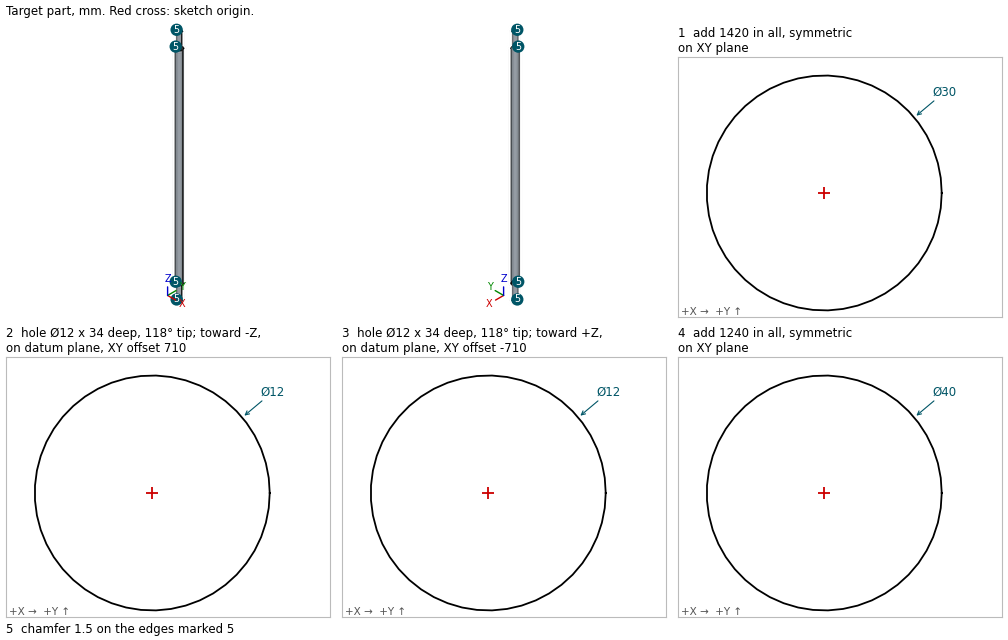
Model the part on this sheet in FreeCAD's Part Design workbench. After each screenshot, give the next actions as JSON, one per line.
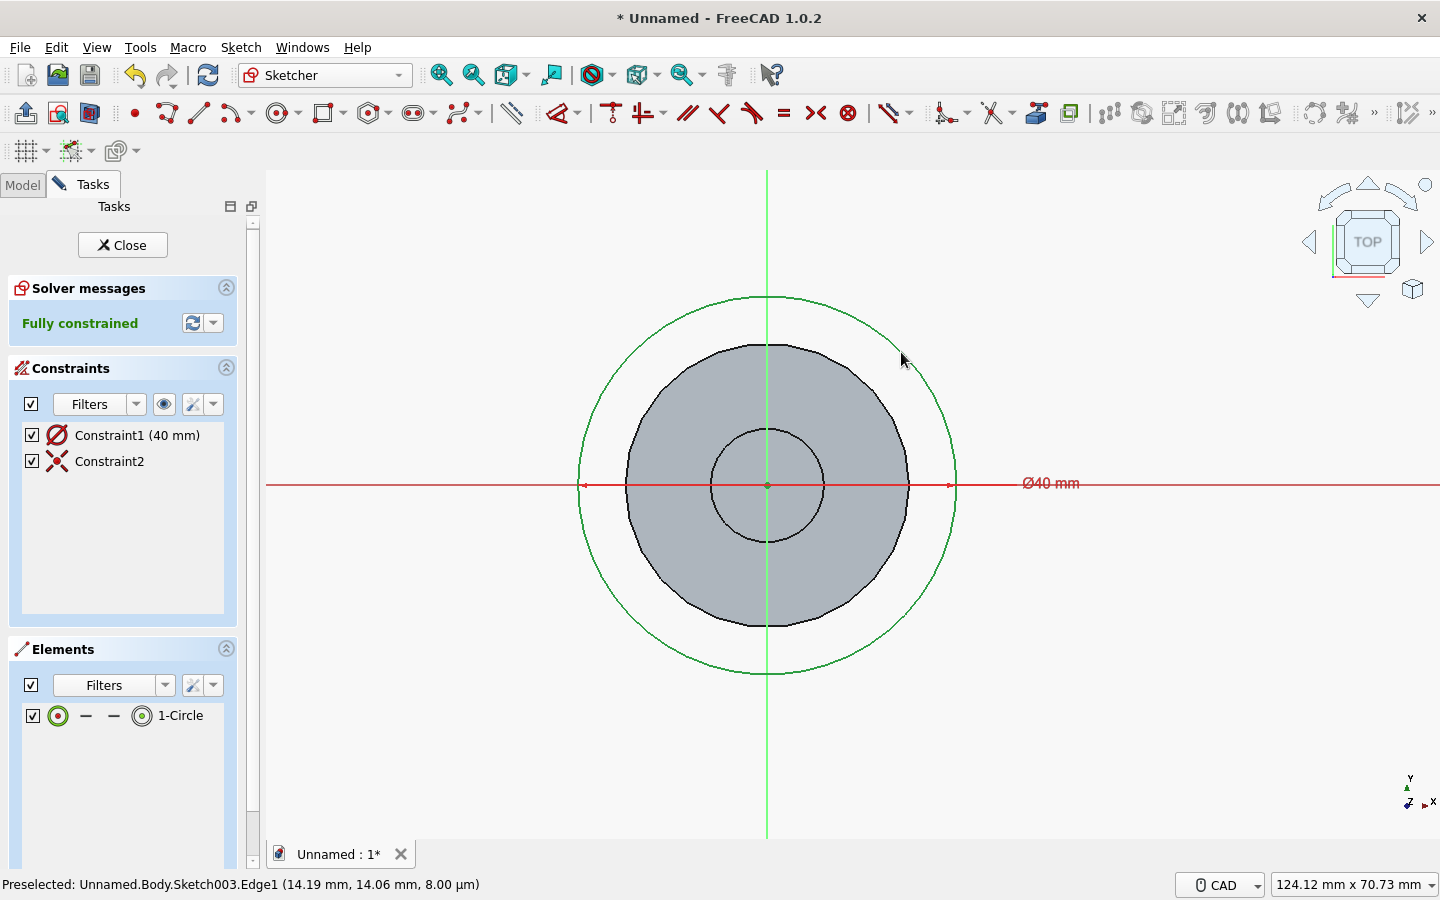
{"action": "left_click", "coordinate": [123, 245]}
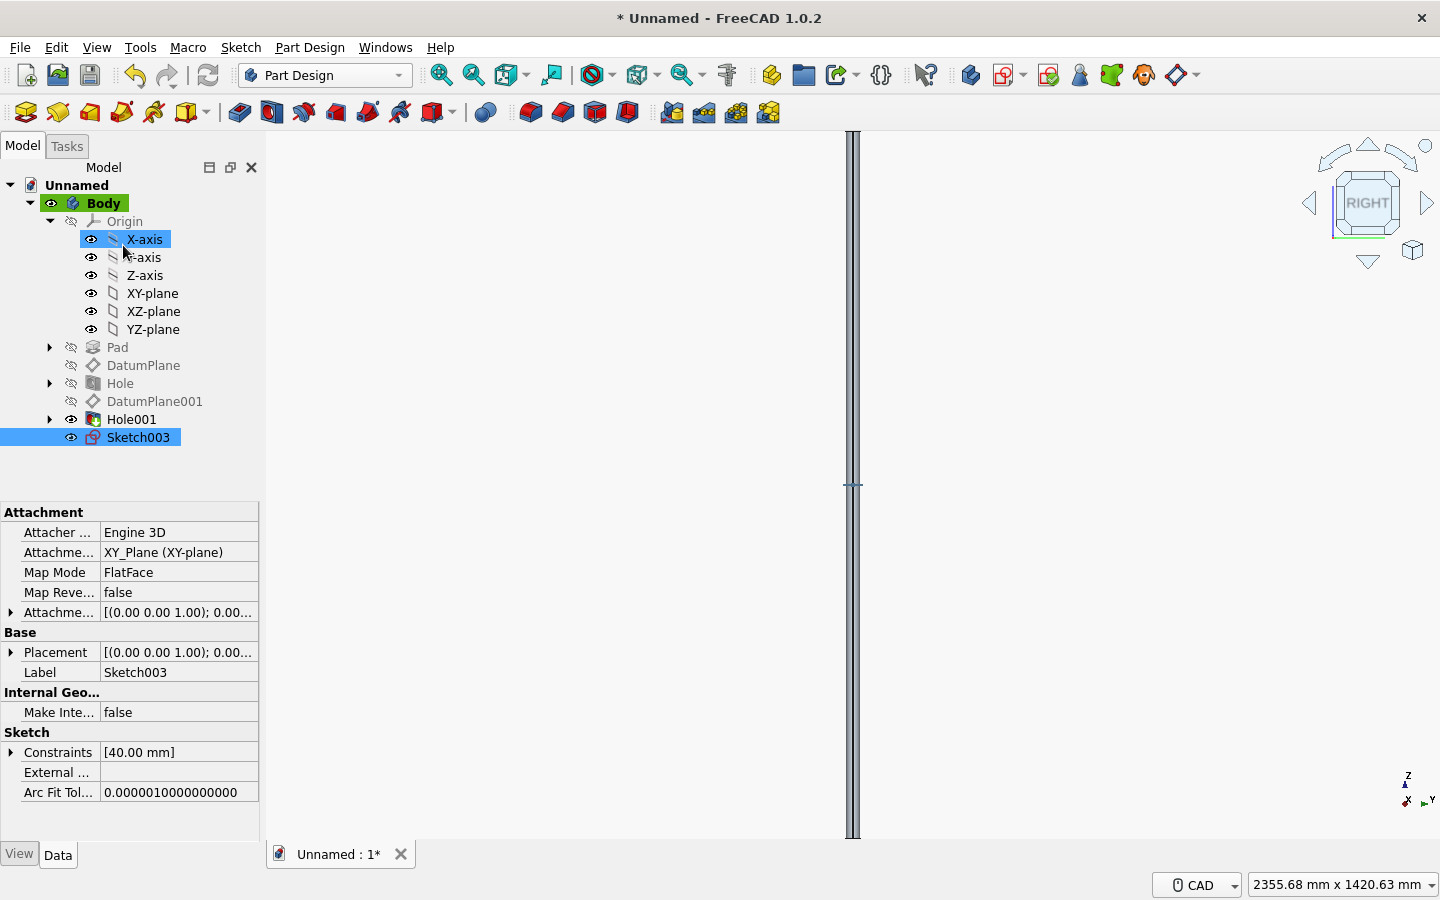
{"action": "left_click", "coordinate": [26, 112]}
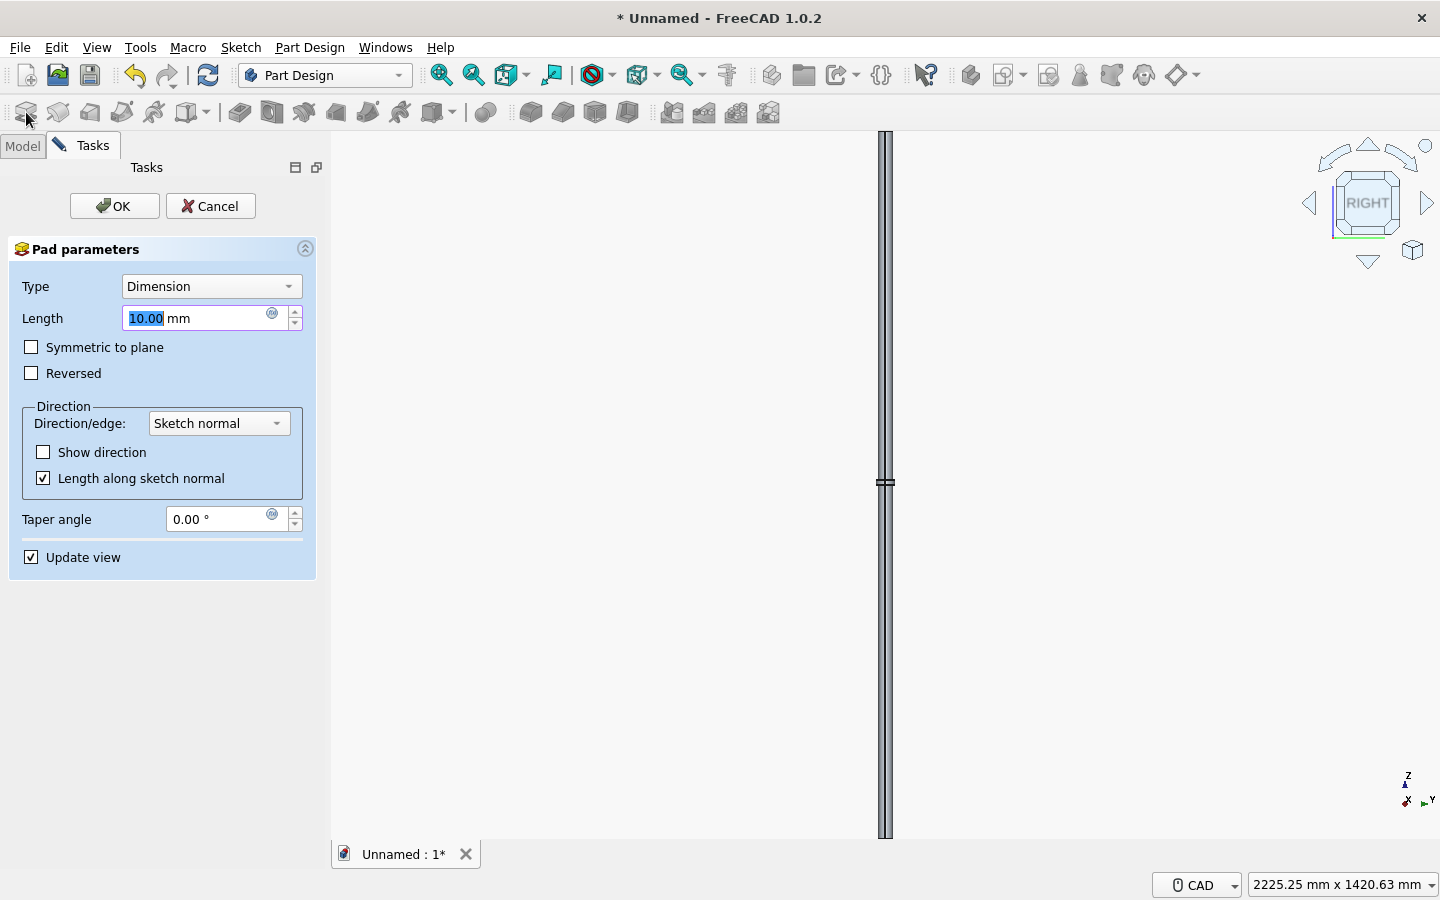
{"action": "type", "text": "1240"}
{"action": "key", "text": "Tab"}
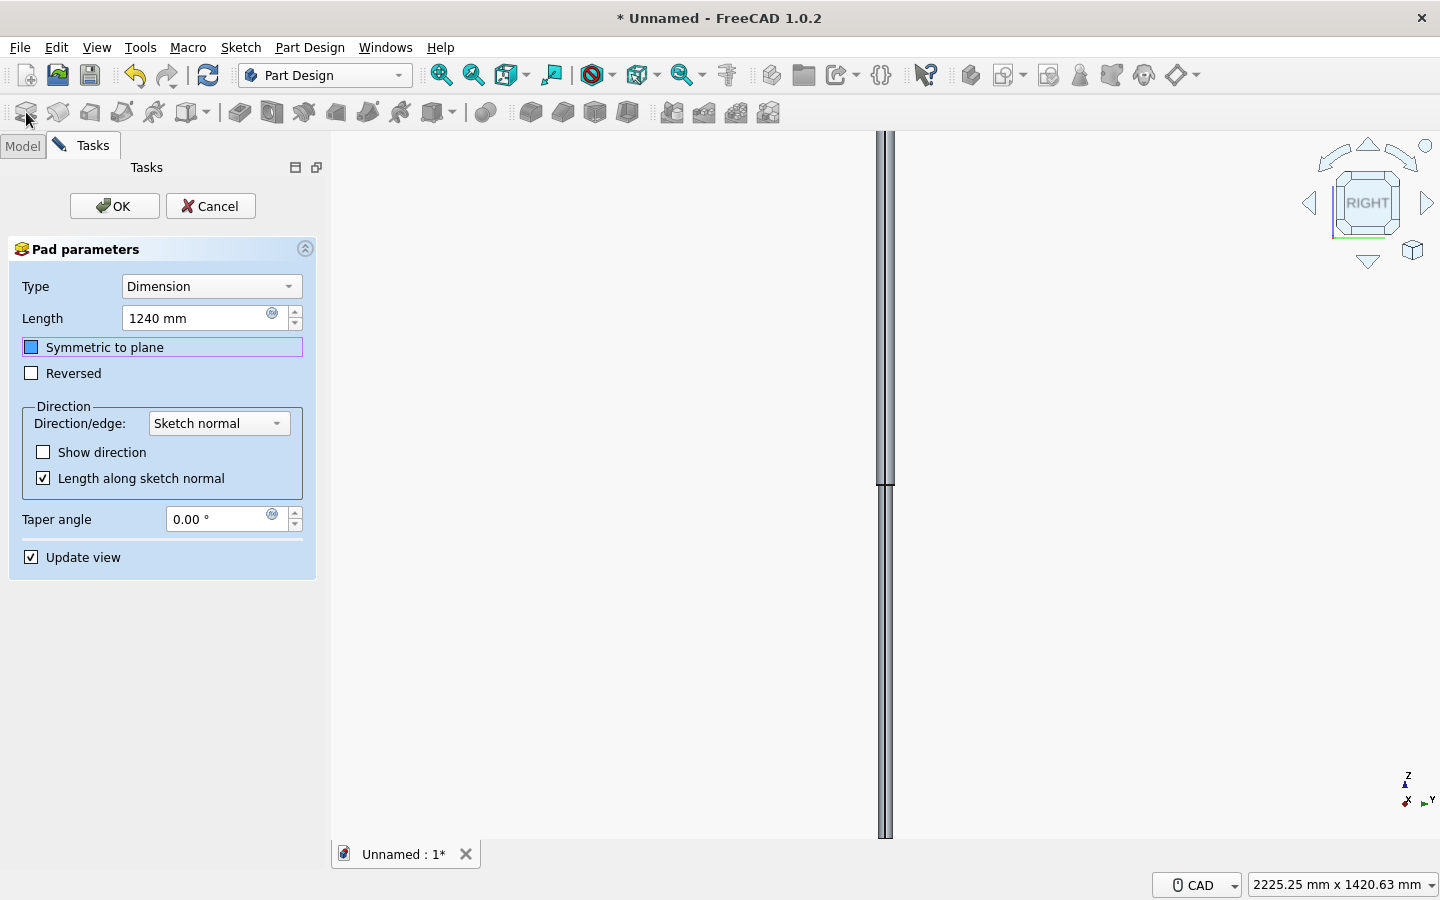
{"action": "left_click", "coordinate": [30, 347]}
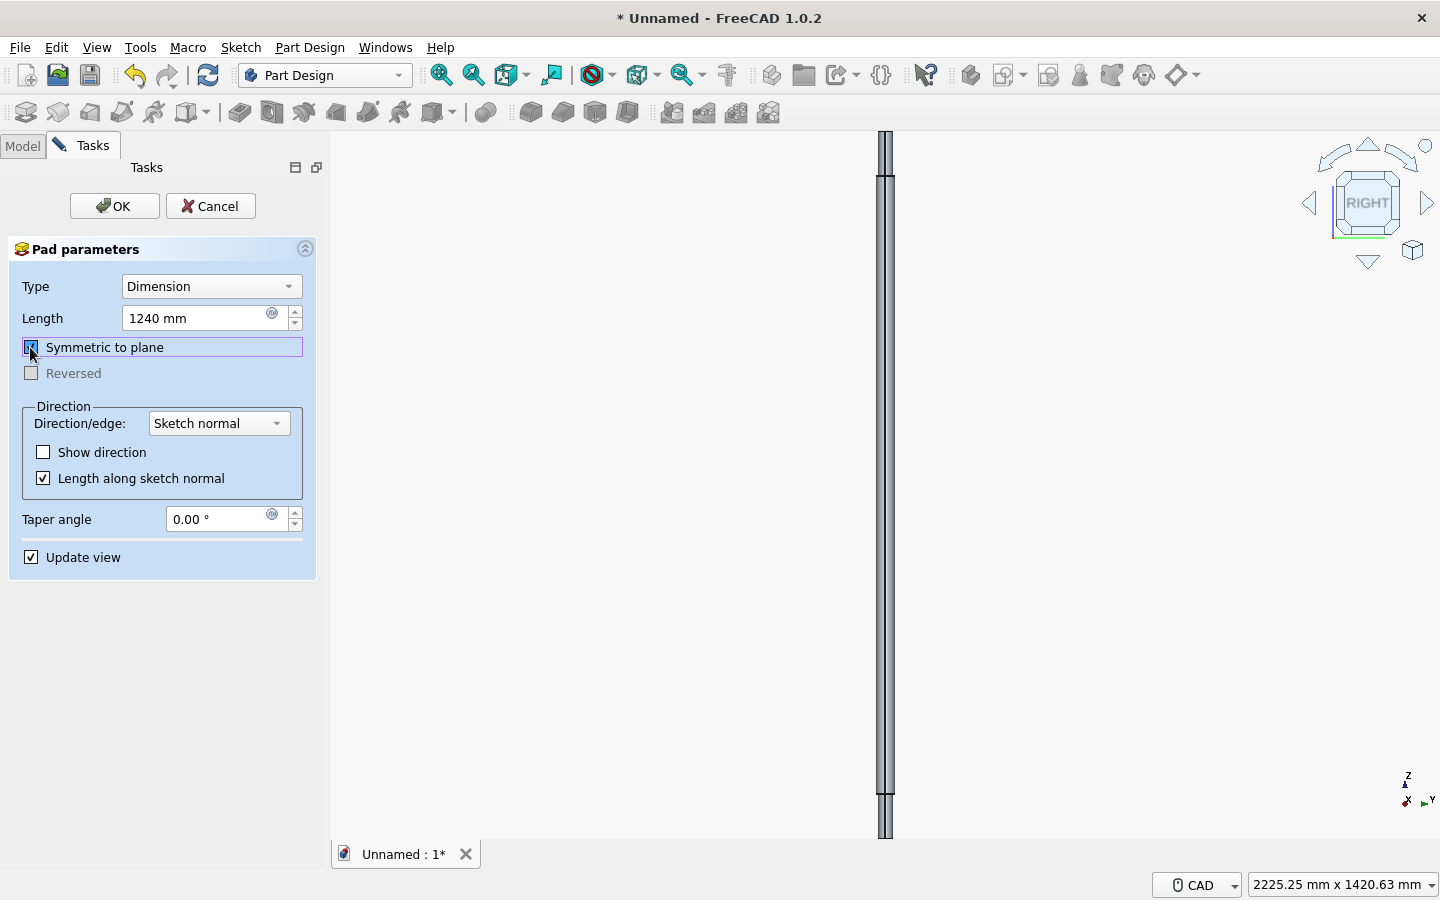
{"action": "left_click", "coordinate": [115, 206]}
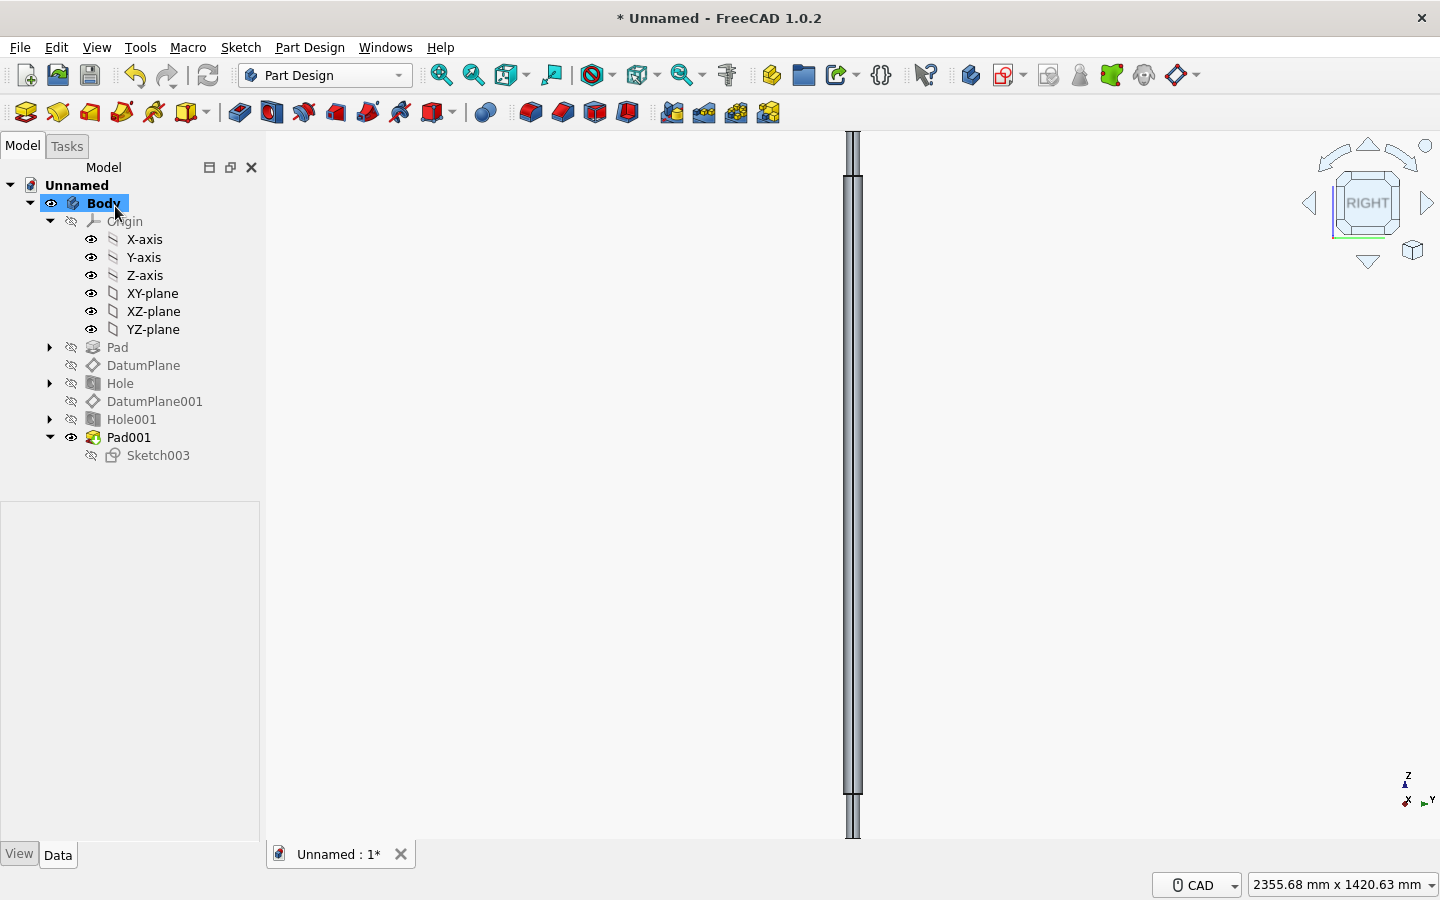
{"action": "left_click", "coordinate": [442, 76]}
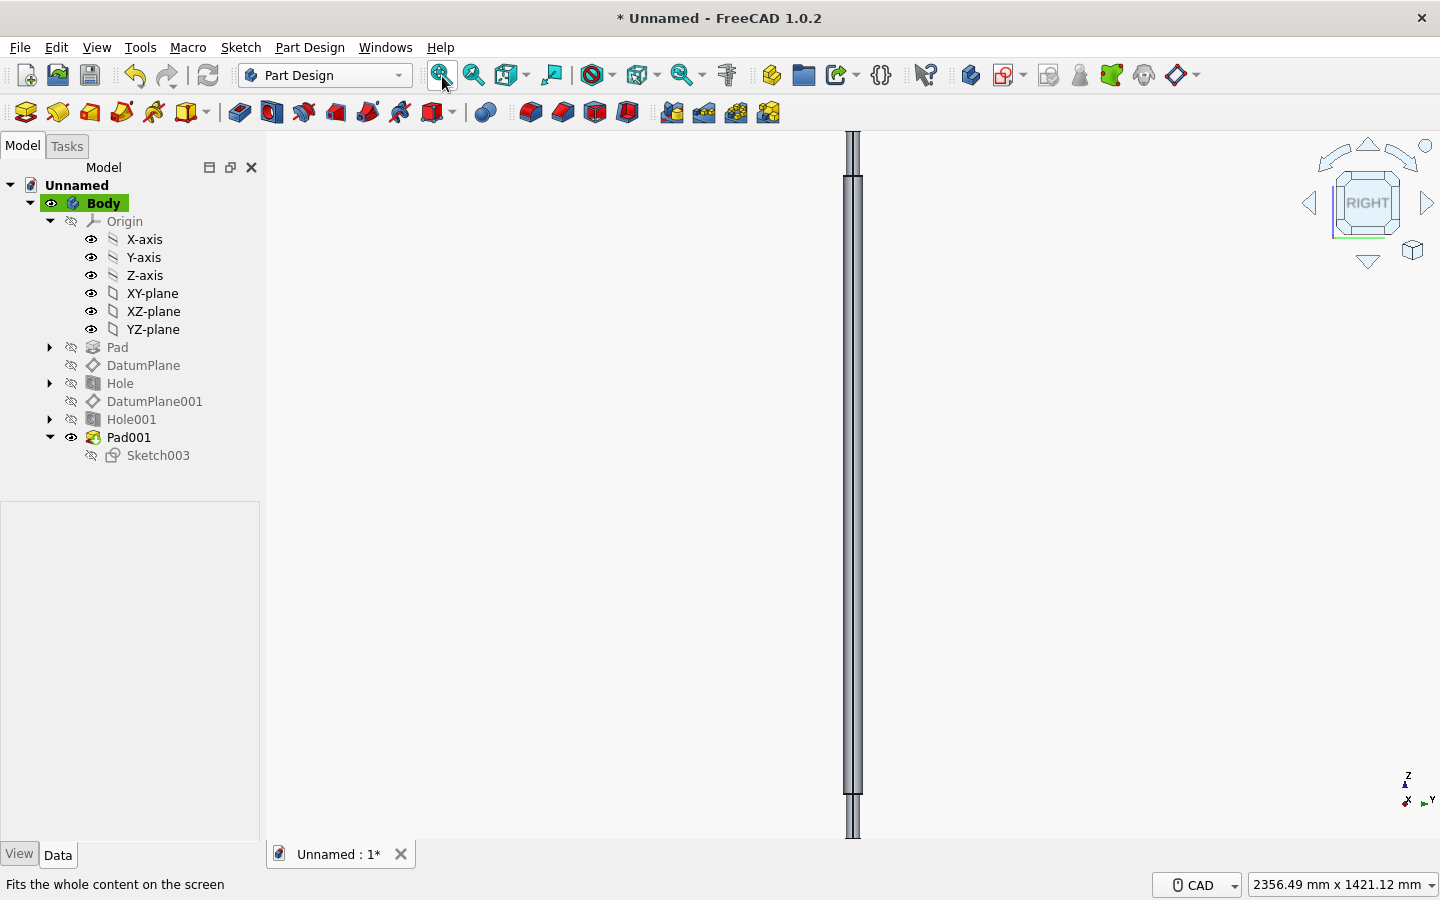
{"action": "left_click", "coordinate": [862, 793]}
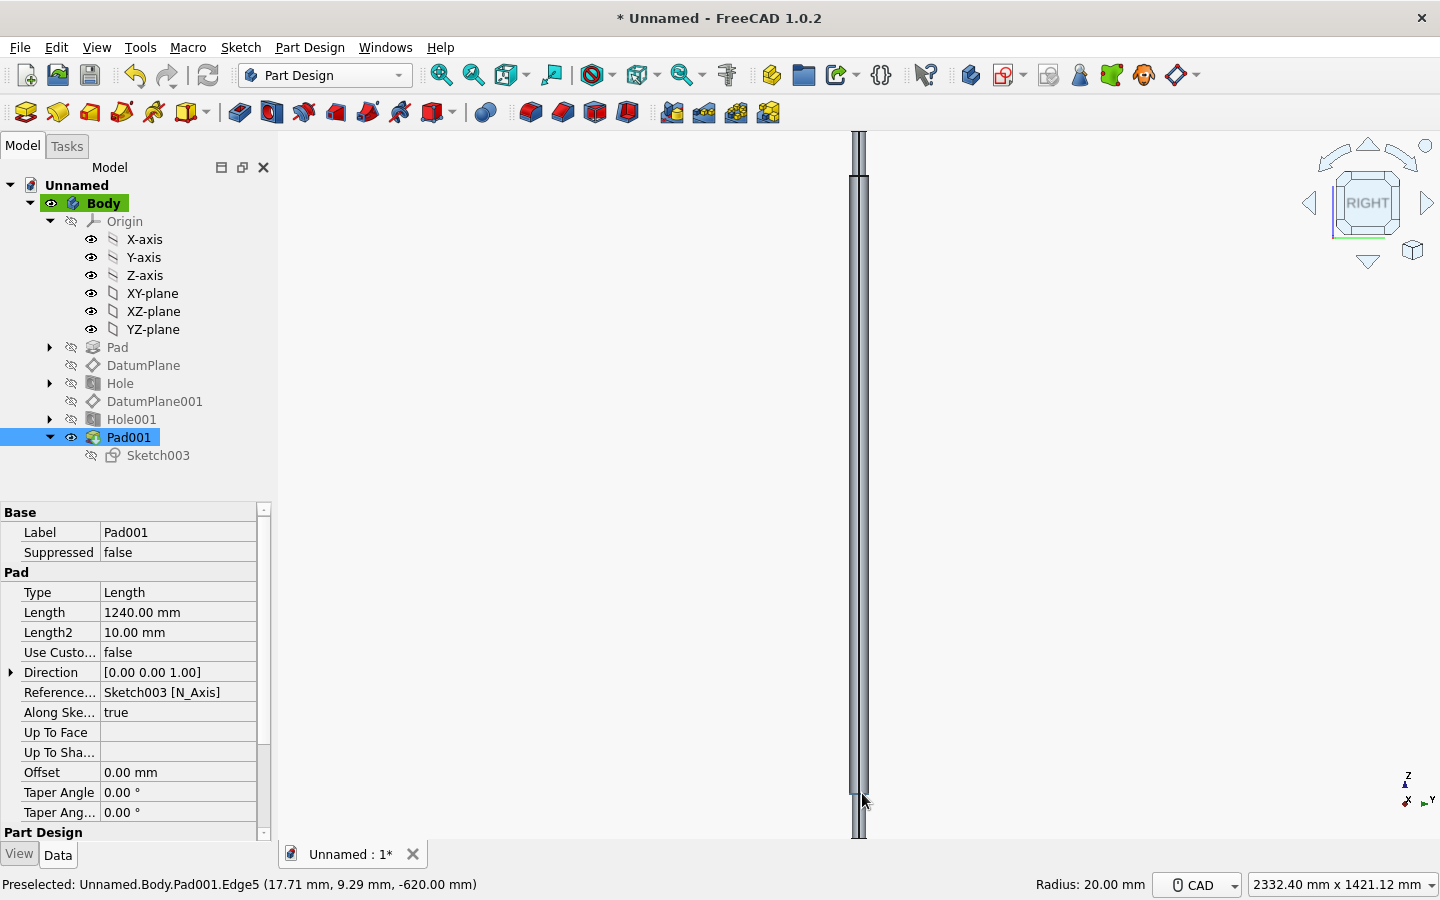
{"action": "left_click", "coordinate": [853, 175], "text": "ctrl"}